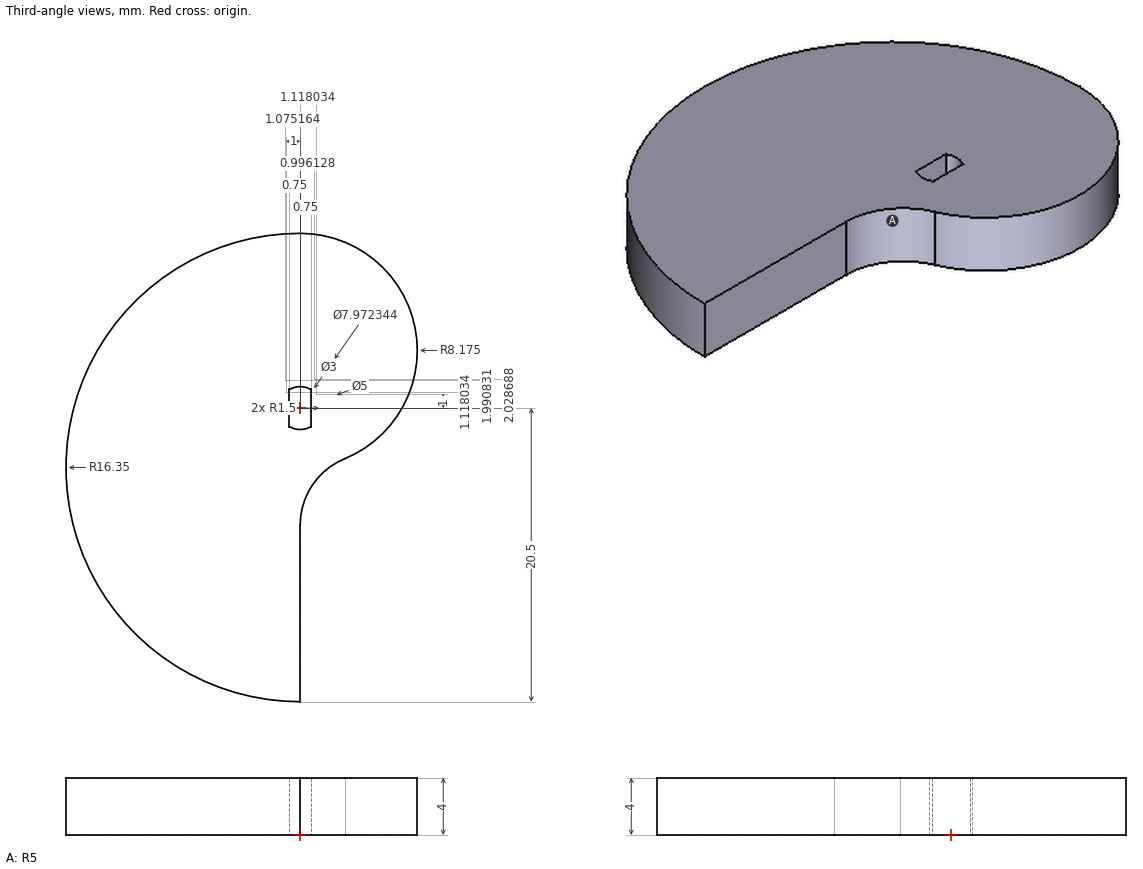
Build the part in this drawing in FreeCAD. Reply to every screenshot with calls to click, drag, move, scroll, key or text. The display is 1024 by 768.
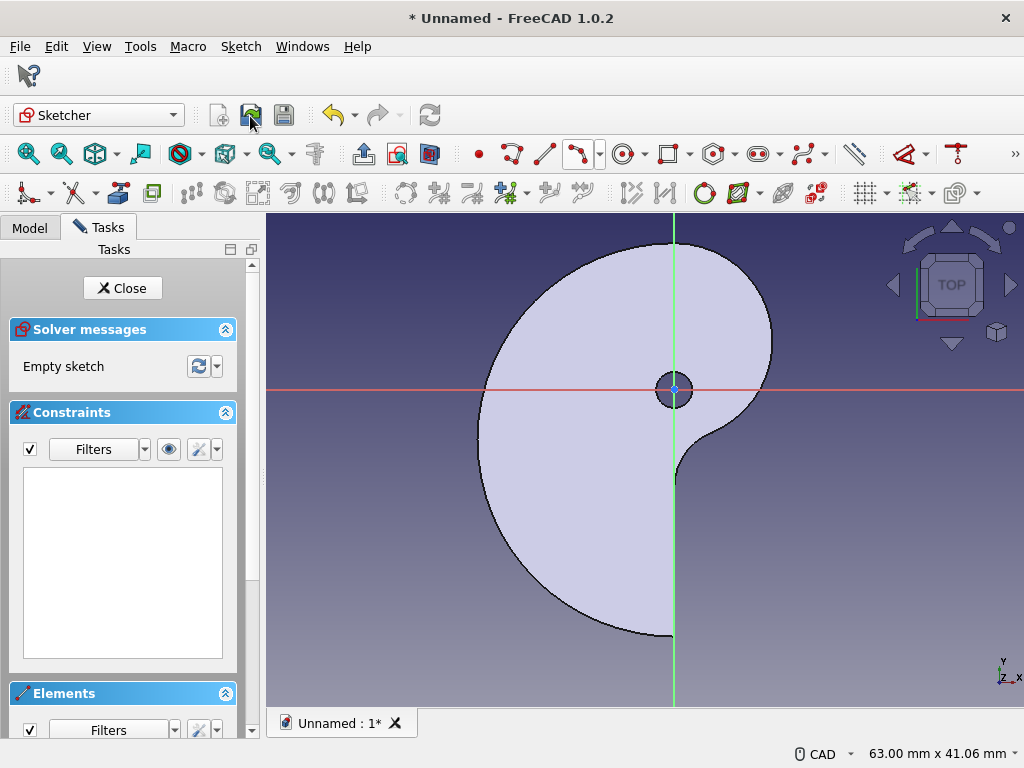
scroll(682, 371, up, 13)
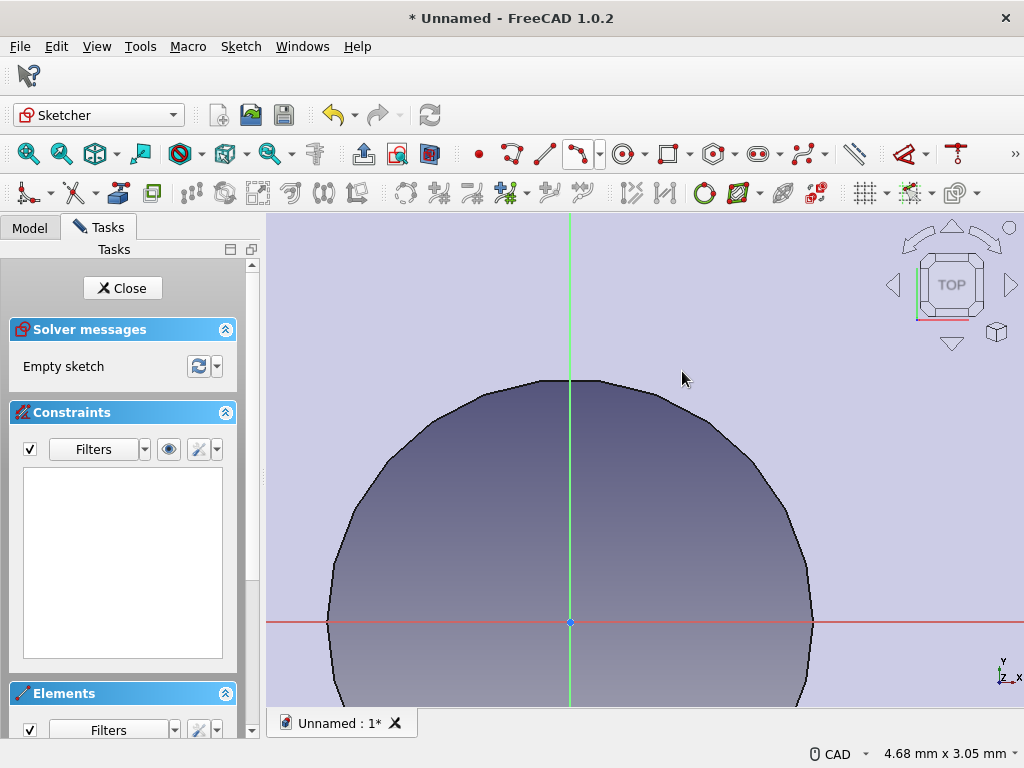
key(g)
key(m)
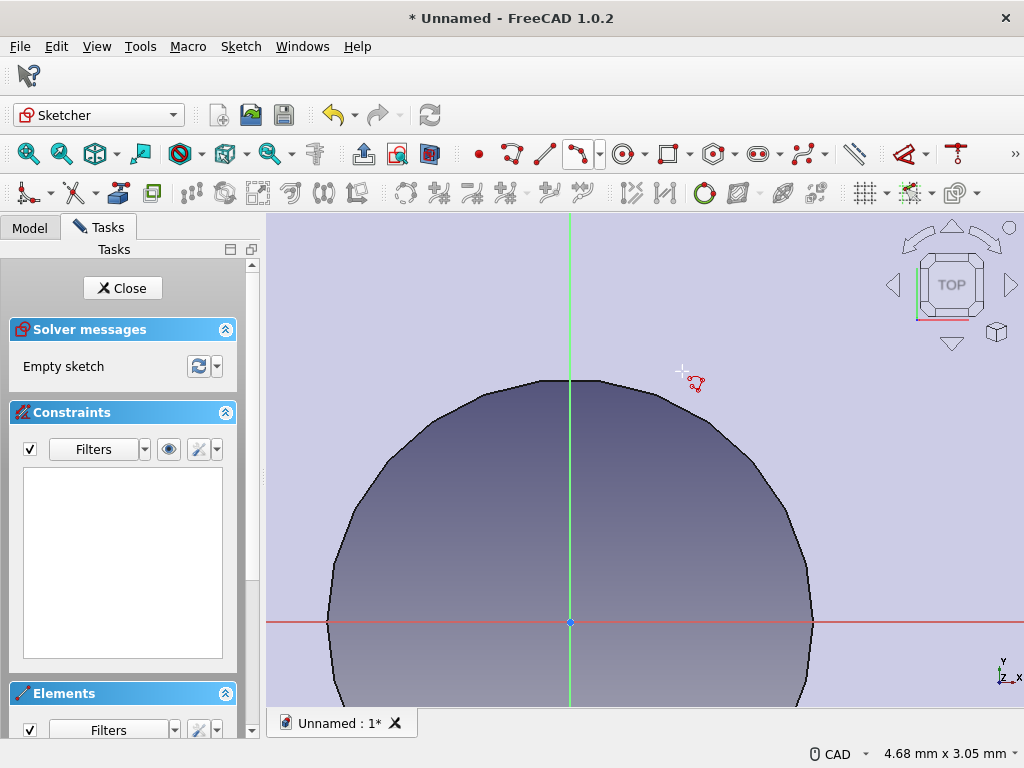
click(570, 622)
click(751, 460)
click(732, 294)
click(396, 311)
click(408, 441)
click(570, 622)
key(Escape)
key(Escape)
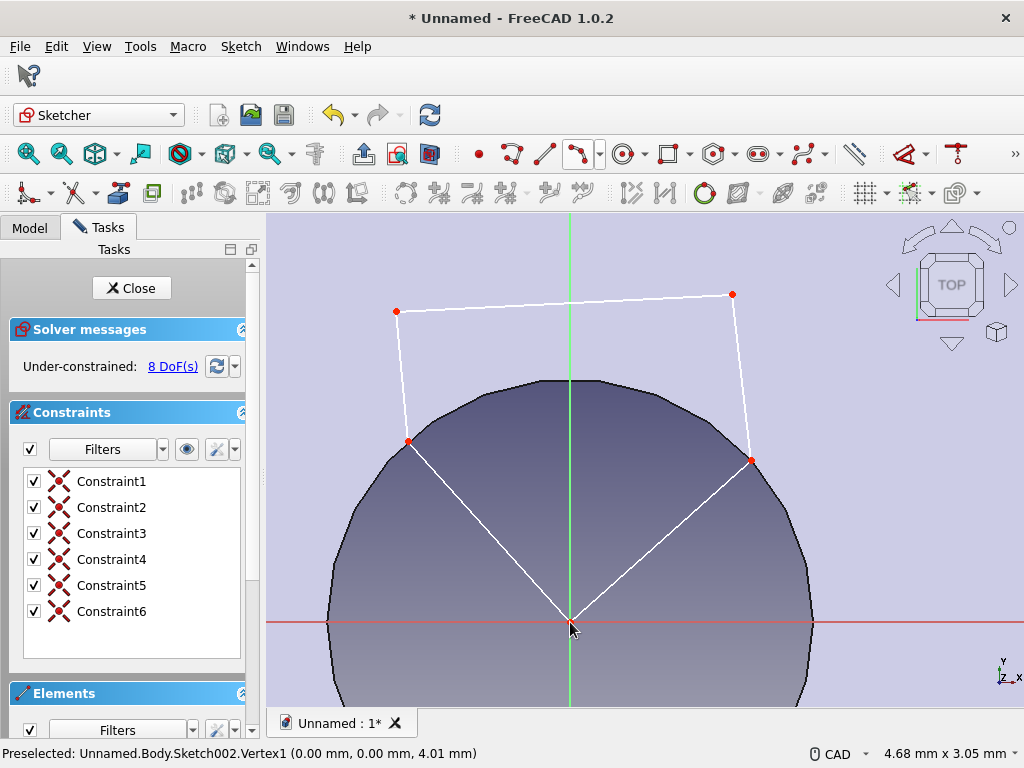
click(904, 154)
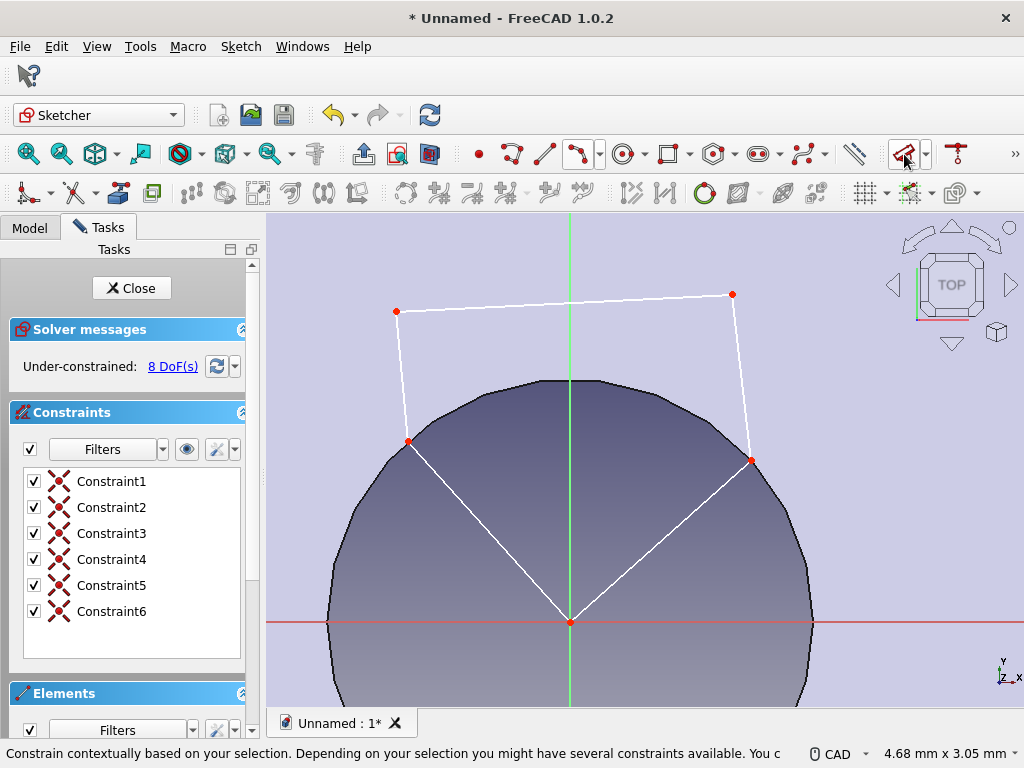
click(751, 461)
click(785, 542)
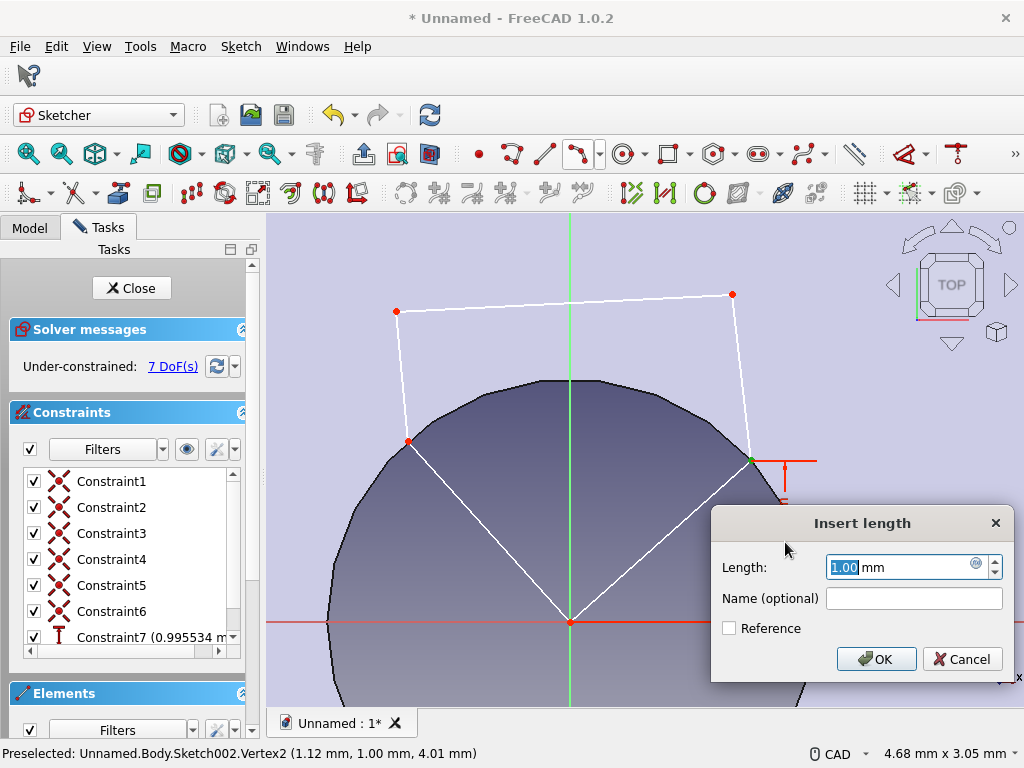
text(1)
key(Return)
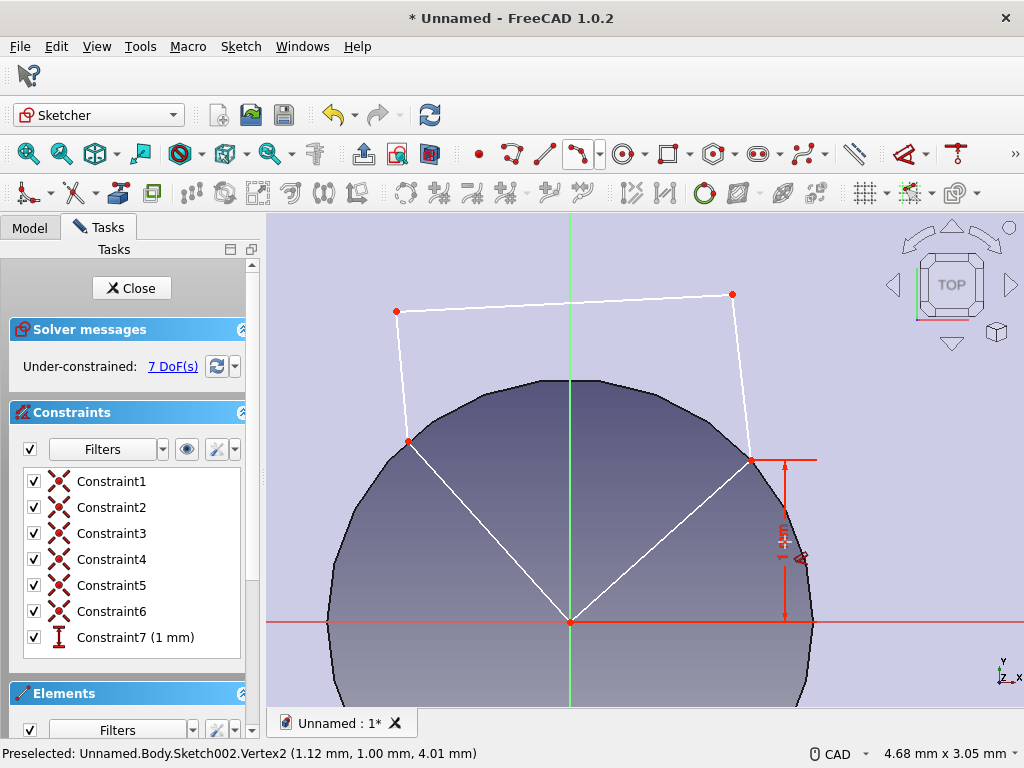
click(408, 442)
click(489, 656)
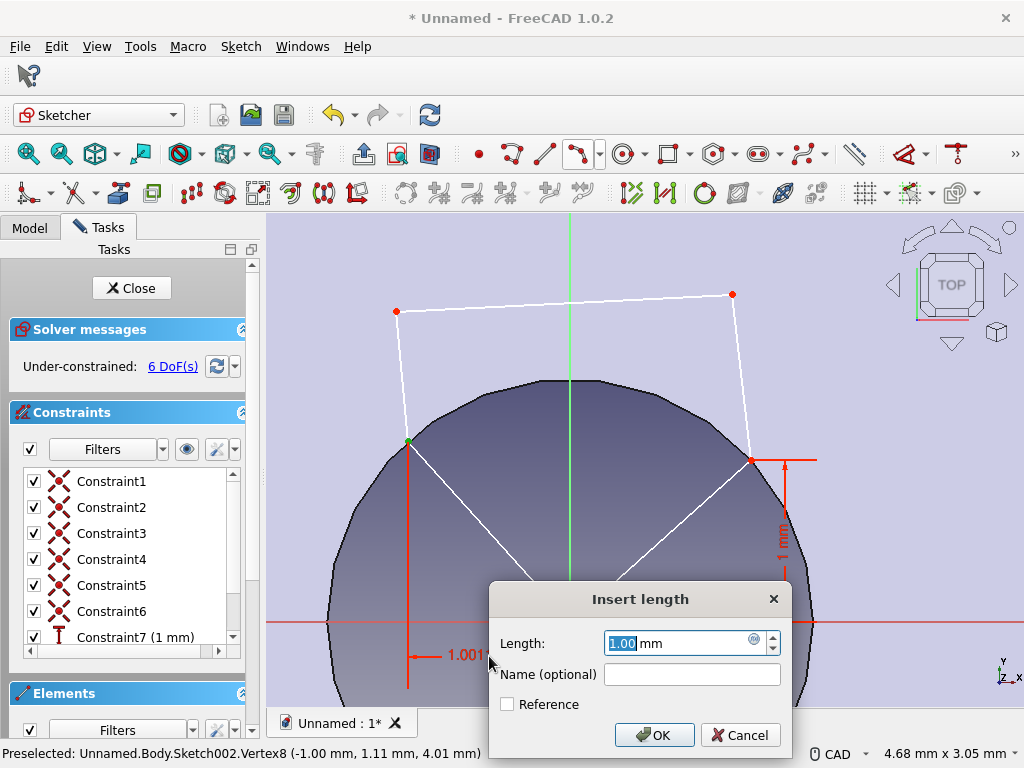
text(1)
key(Return)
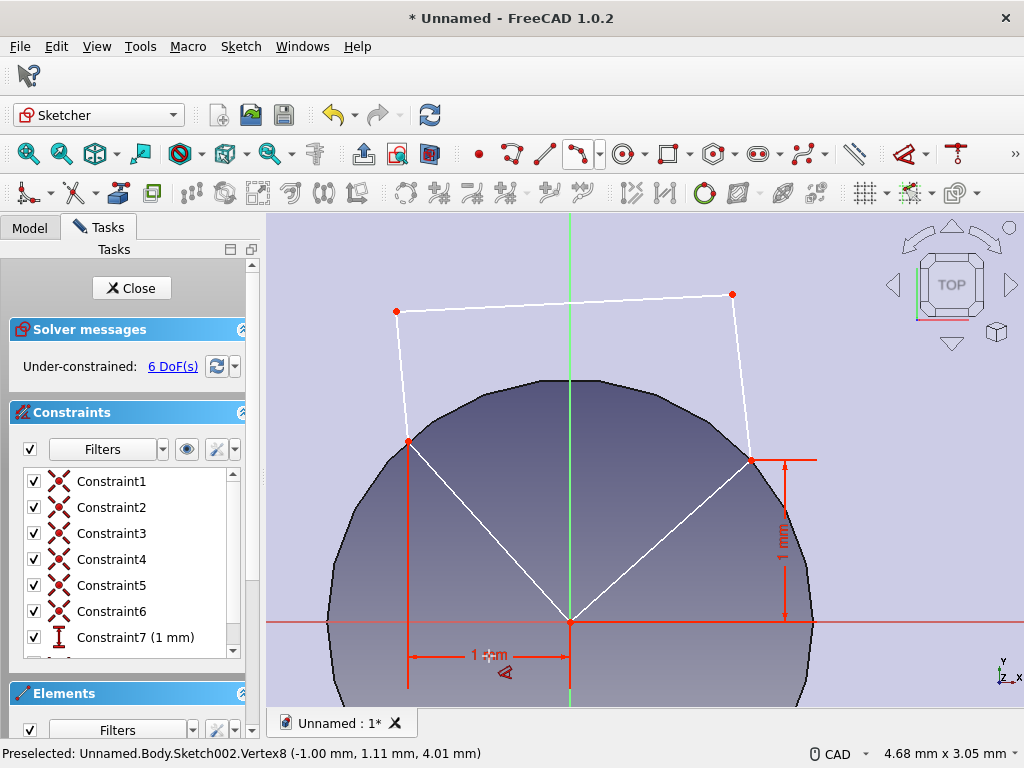
click(751, 460)
click(661, 656)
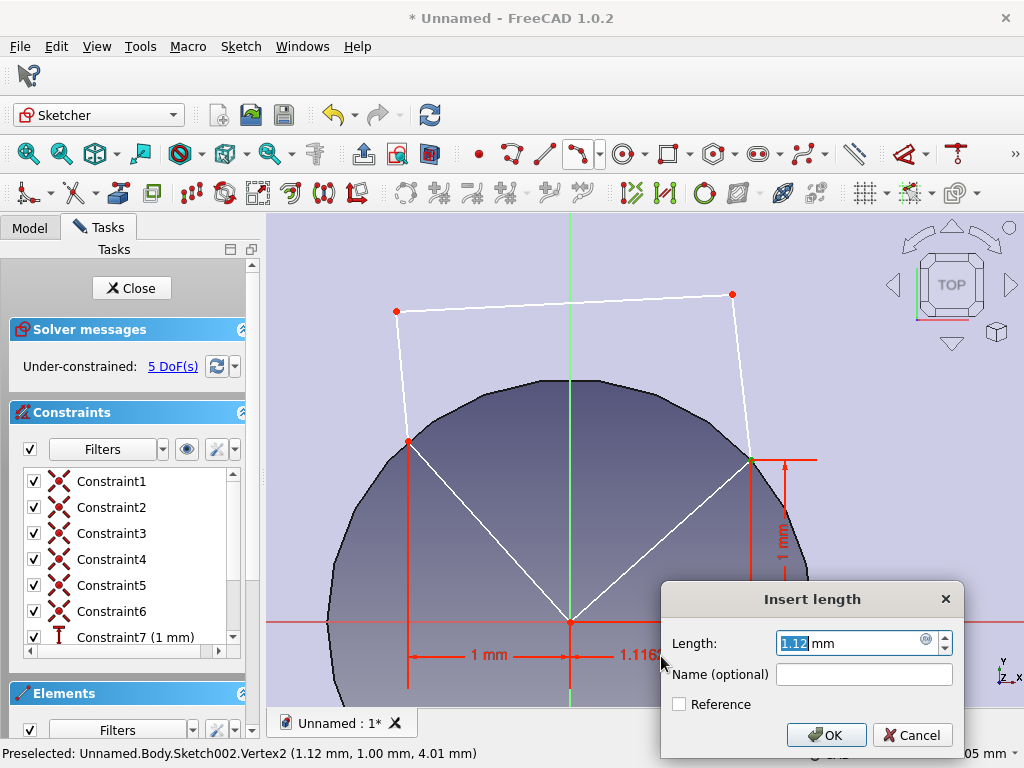
text(1.118034)
key(Return)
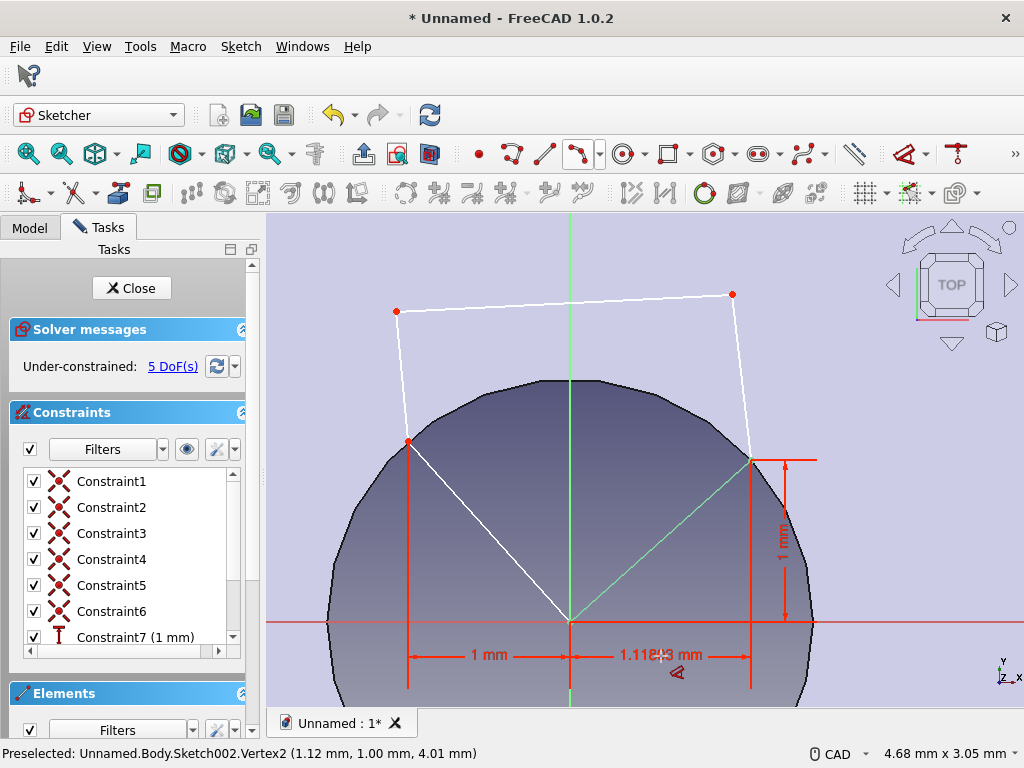
click(732, 295)
click(651, 261)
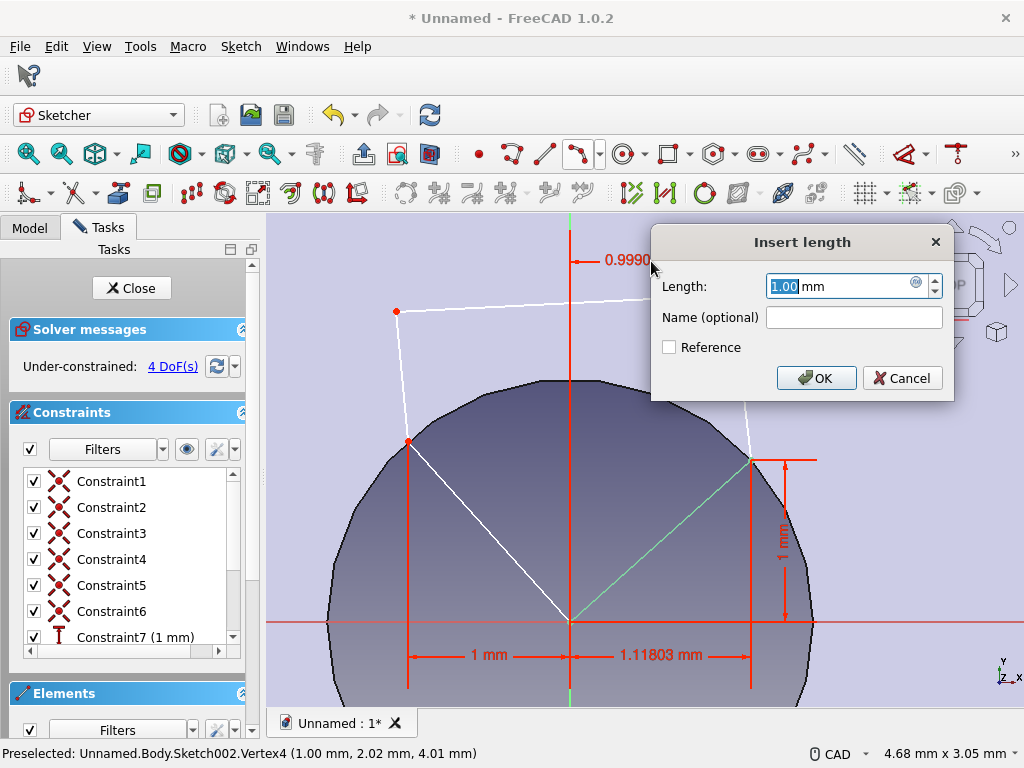
text(0.996128)
key(Return)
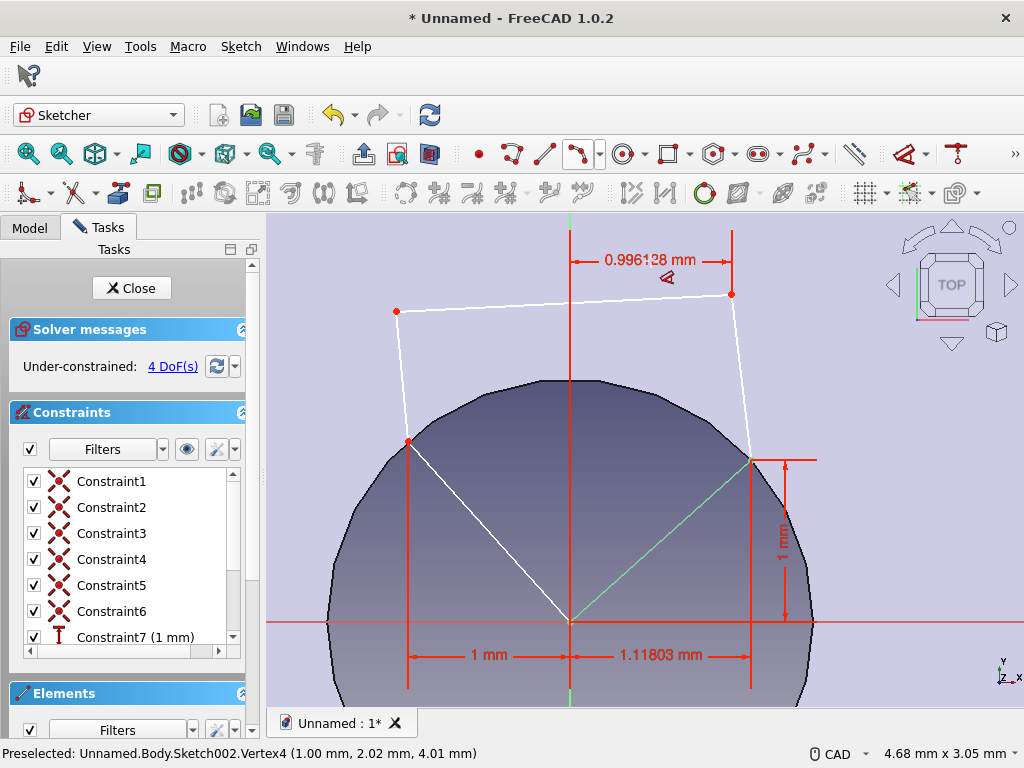
click(732, 295)
click(766, 459)